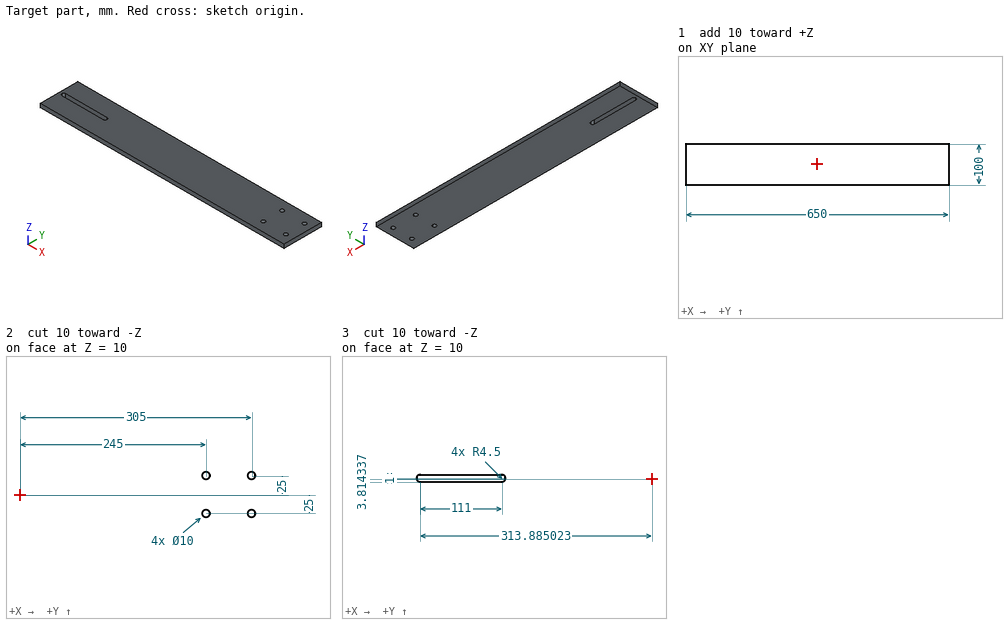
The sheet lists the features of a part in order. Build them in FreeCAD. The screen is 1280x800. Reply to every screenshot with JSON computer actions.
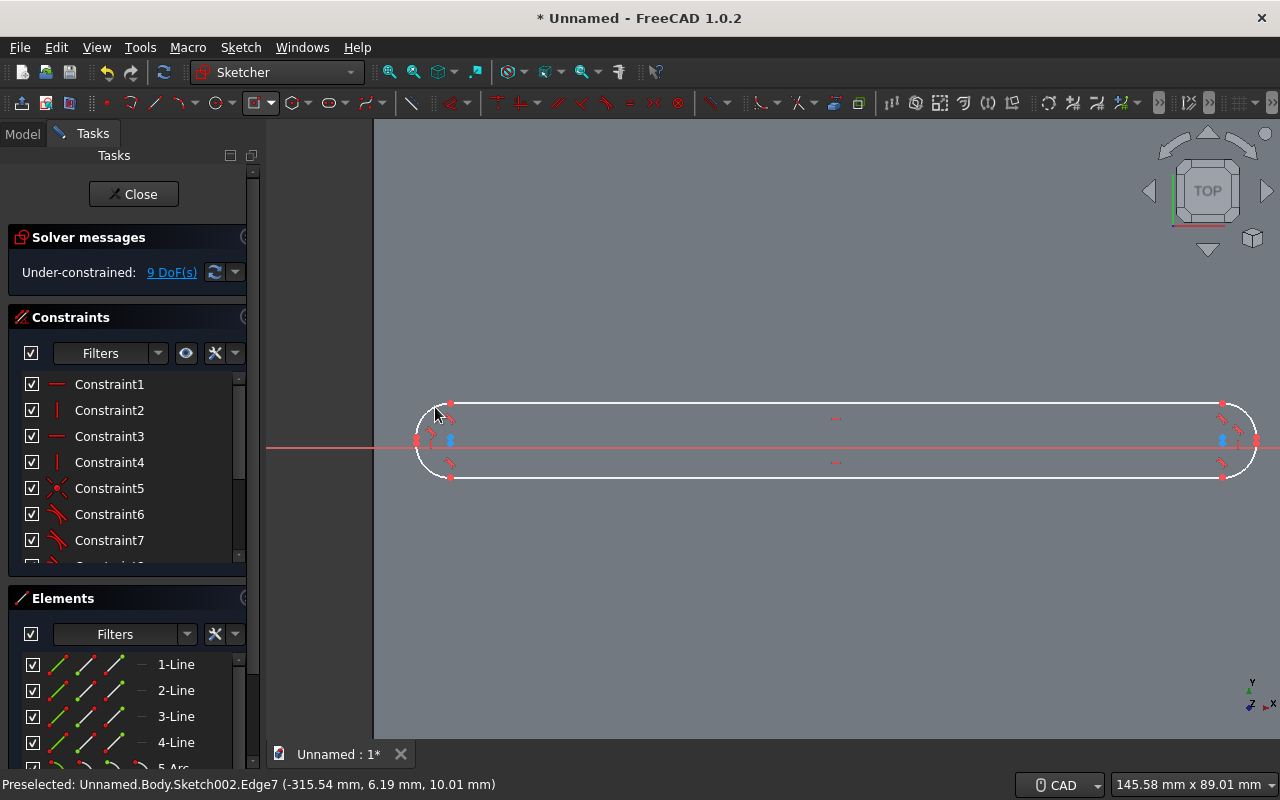
{"action": "scroll", "coordinate": [416, 441], "scroll_direction": "up", "scroll_amount": 8}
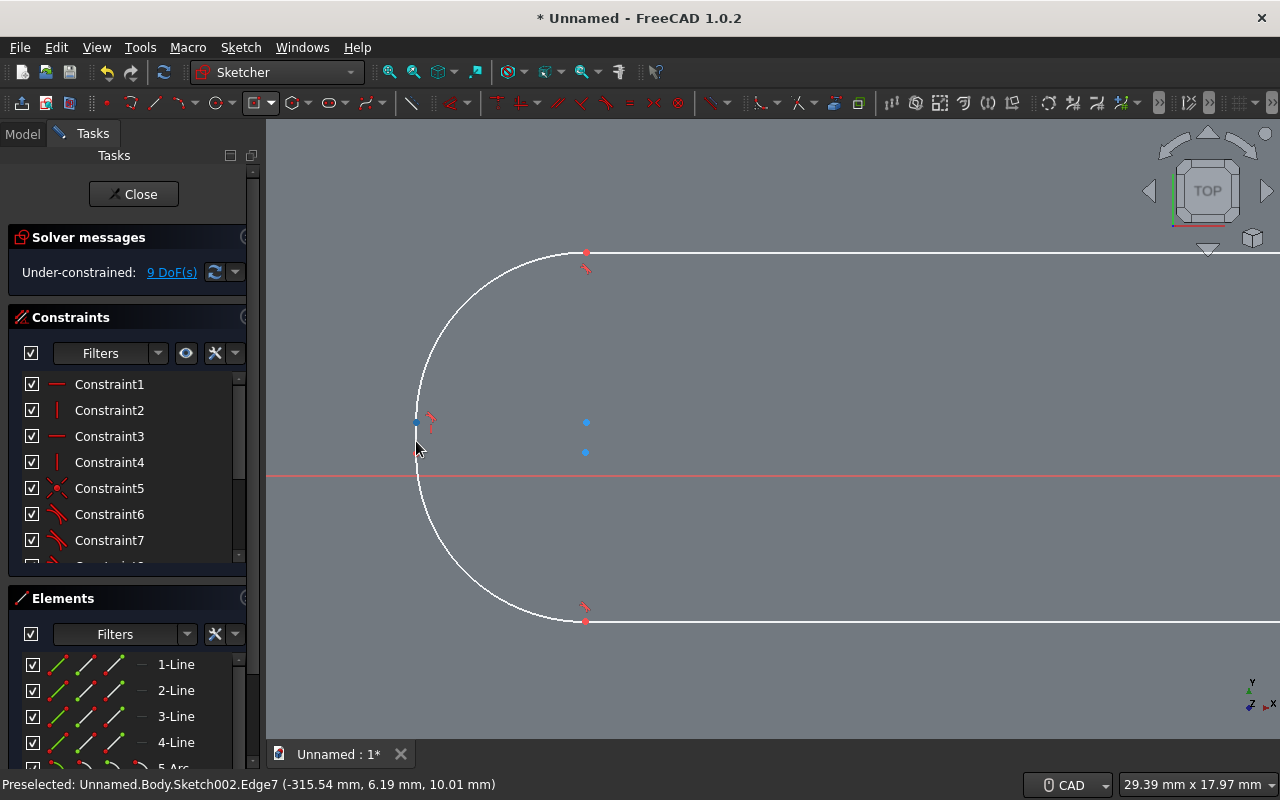
{"action": "left_click", "coordinate": [416, 438]}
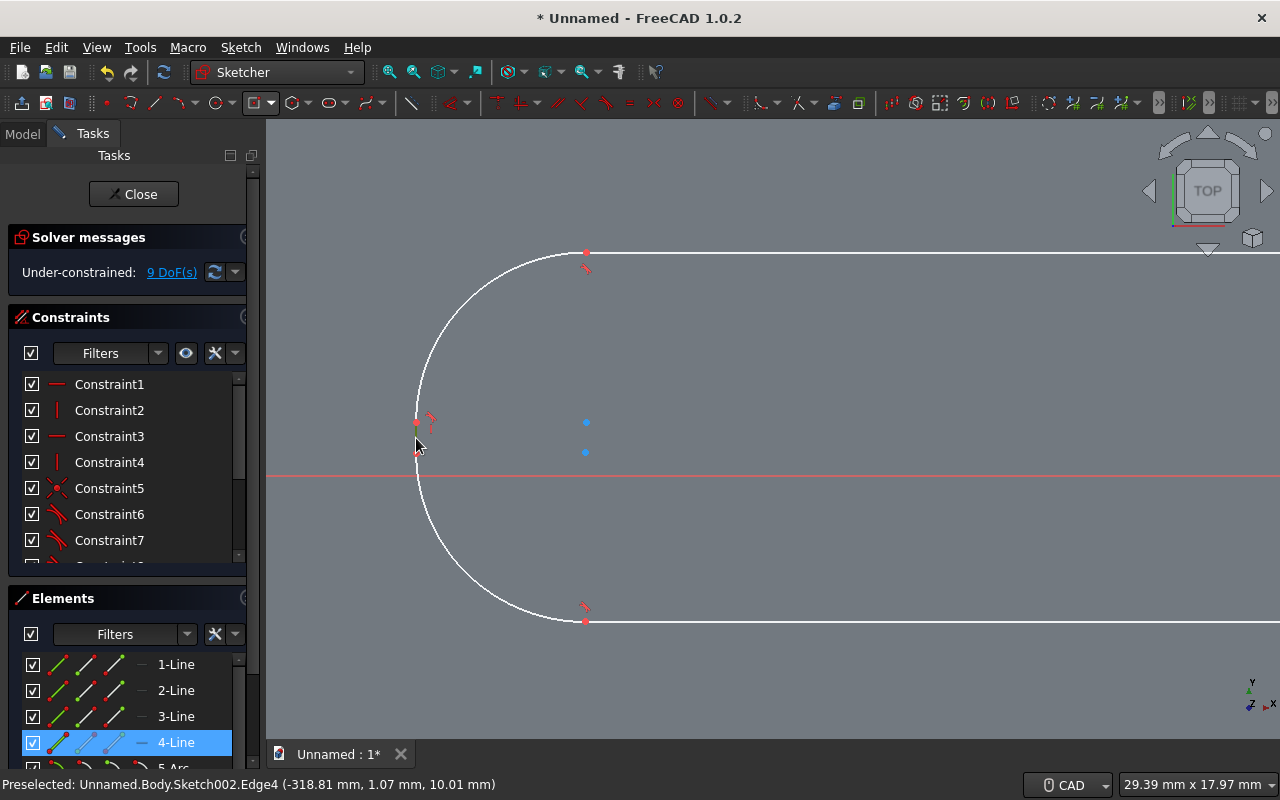
{"action": "scroll", "coordinate": [423, 428], "scroll_direction": "down", "scroll_amount": 10}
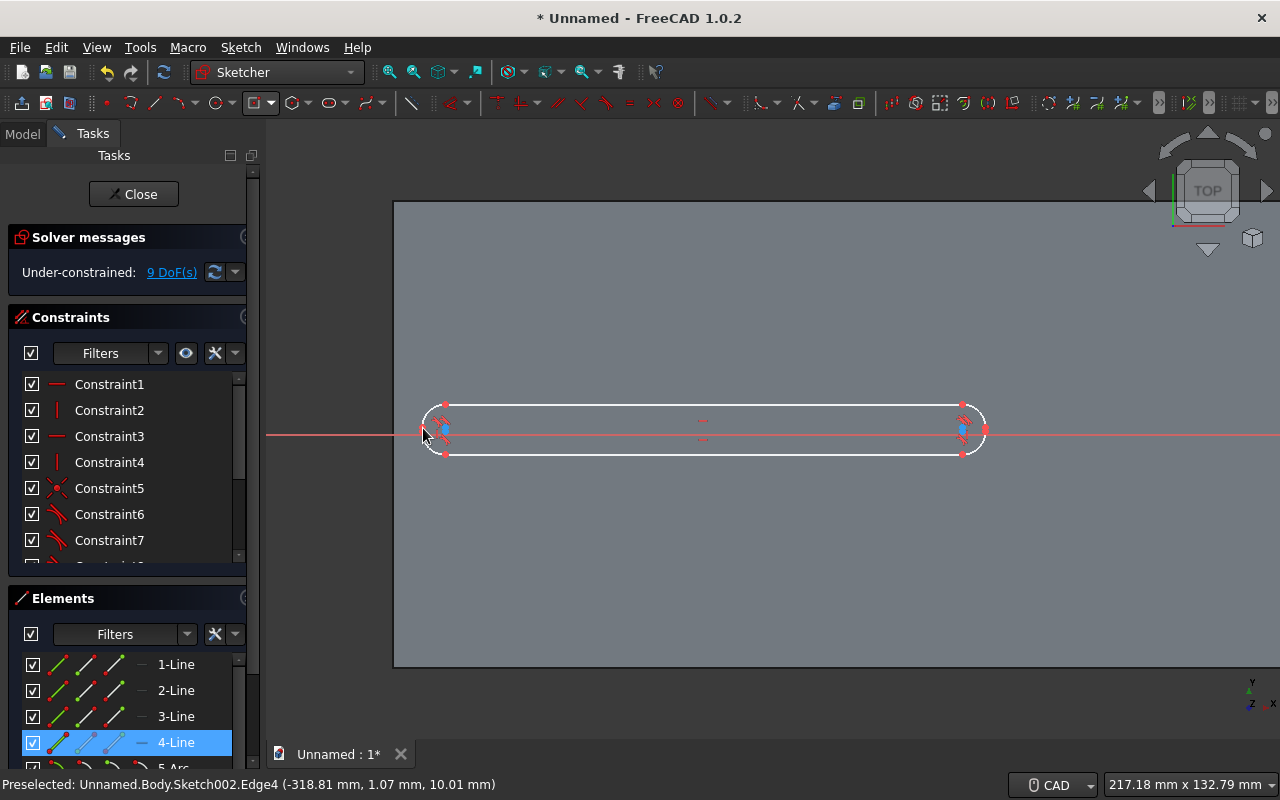
{"action": "scroll", "coordinate": [425, 442], "scroll_direction": "up", "scroll_amount": 4}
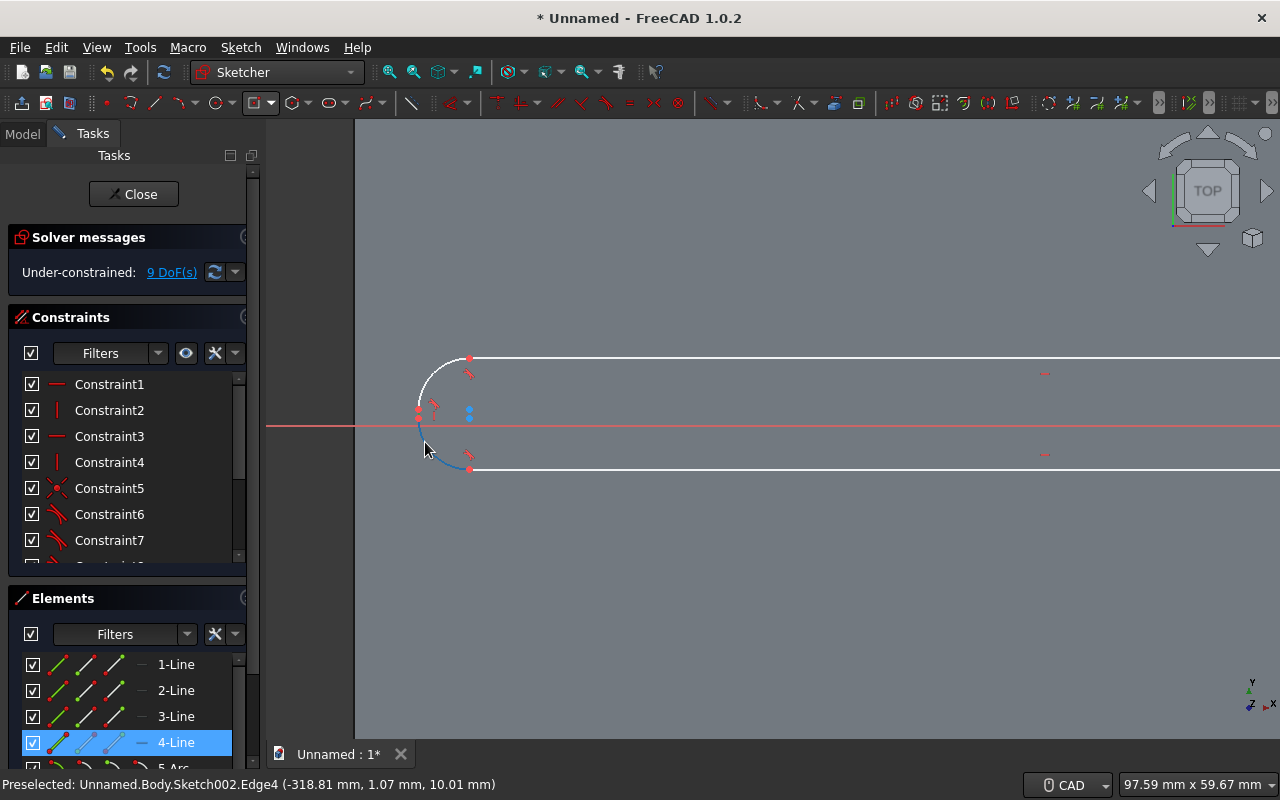
{"action": "left_click", "coordinate": [424, 442]}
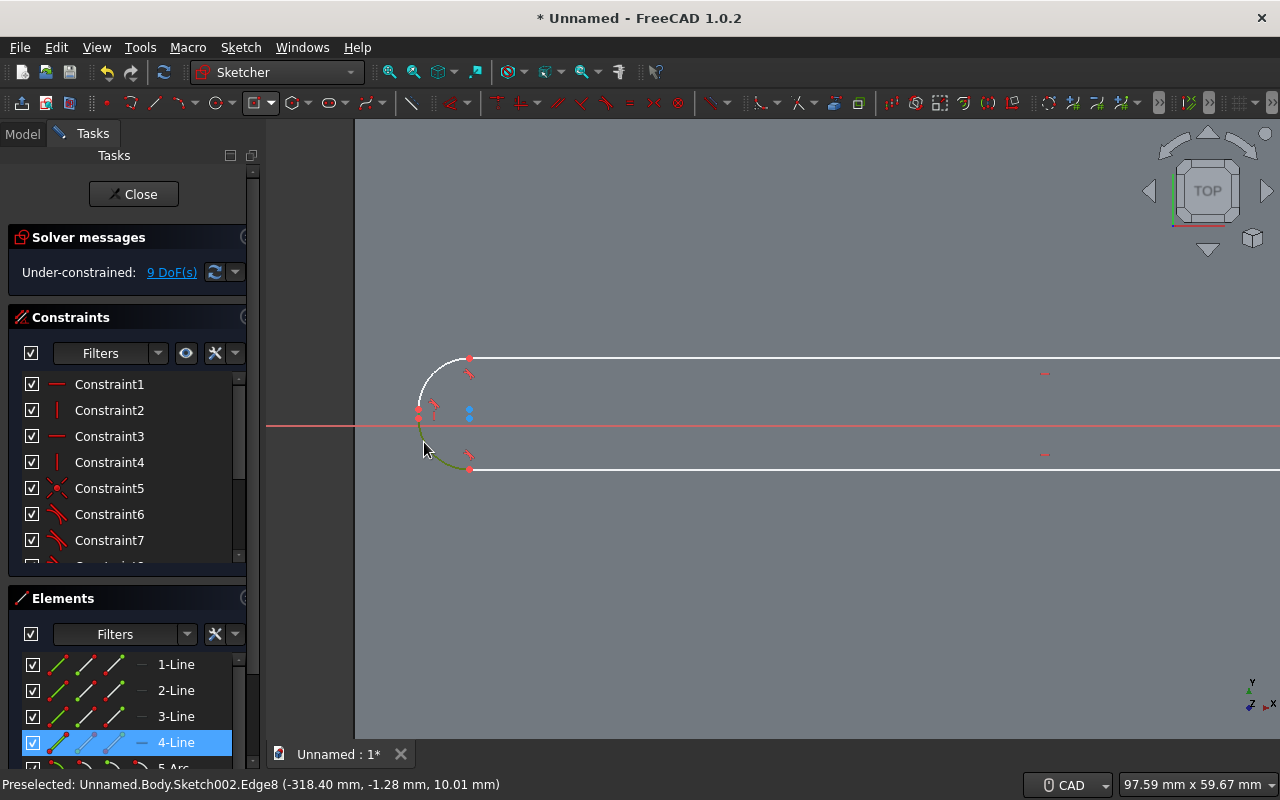
{"action": "key", "text": "t"}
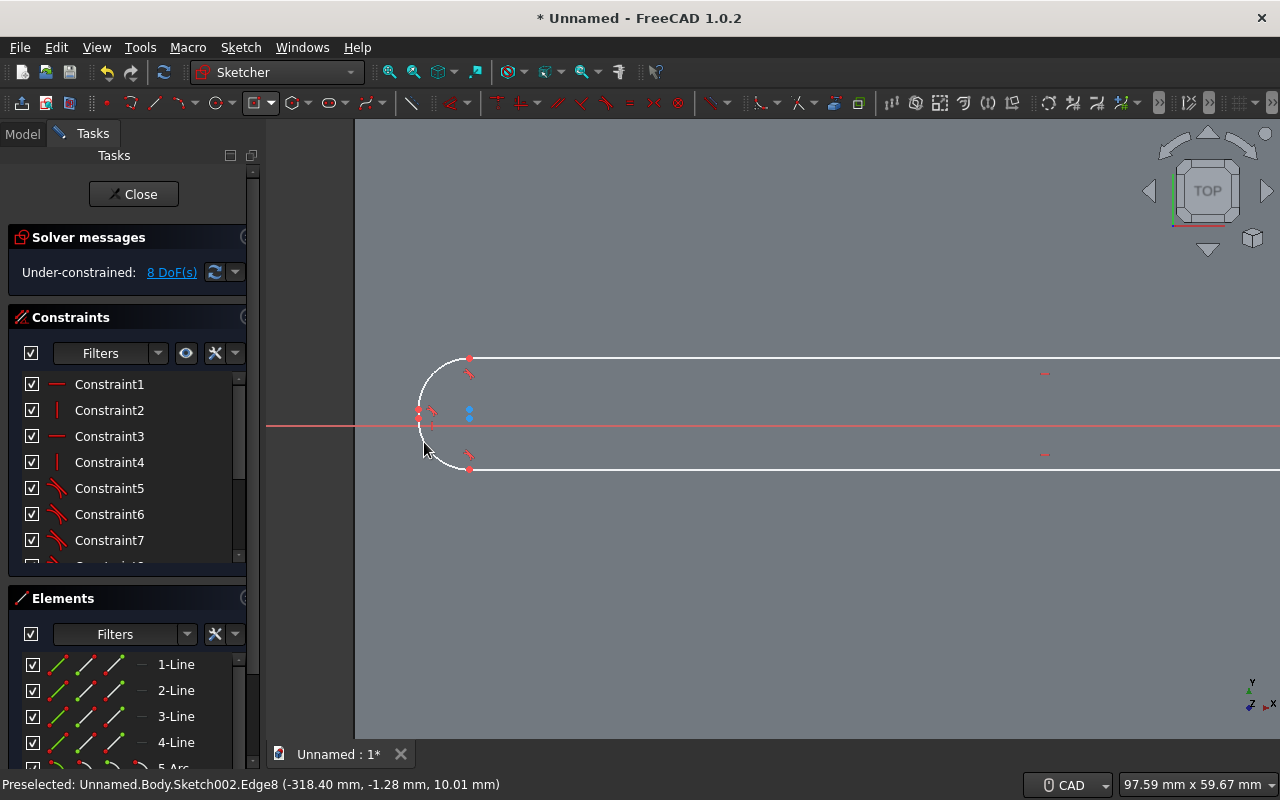
{"action": "scroll", "coordinate": [425, 442], "scroll_direction": "down", "scroll_amount": 4}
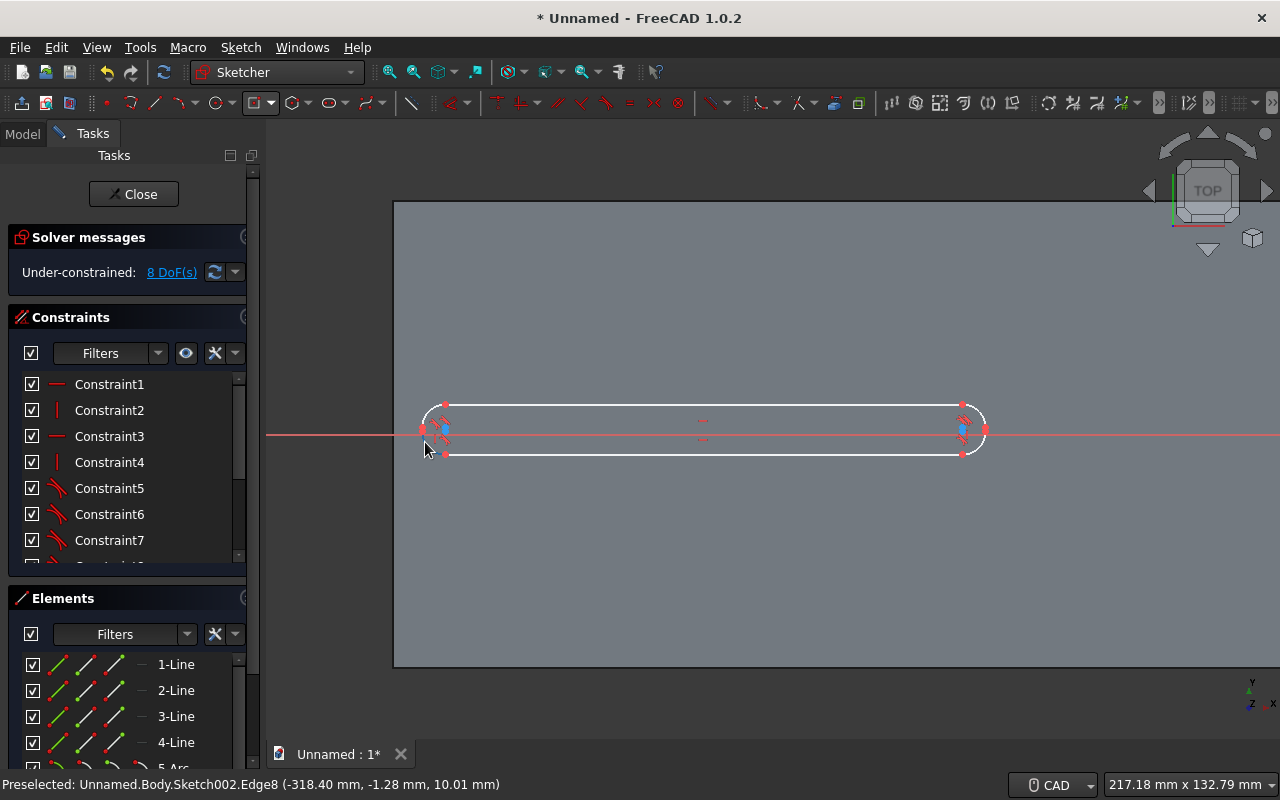
{"action": "scroll", "coordinate": [973, 452], "scroll_direction": "up", "scroll_amount": 2}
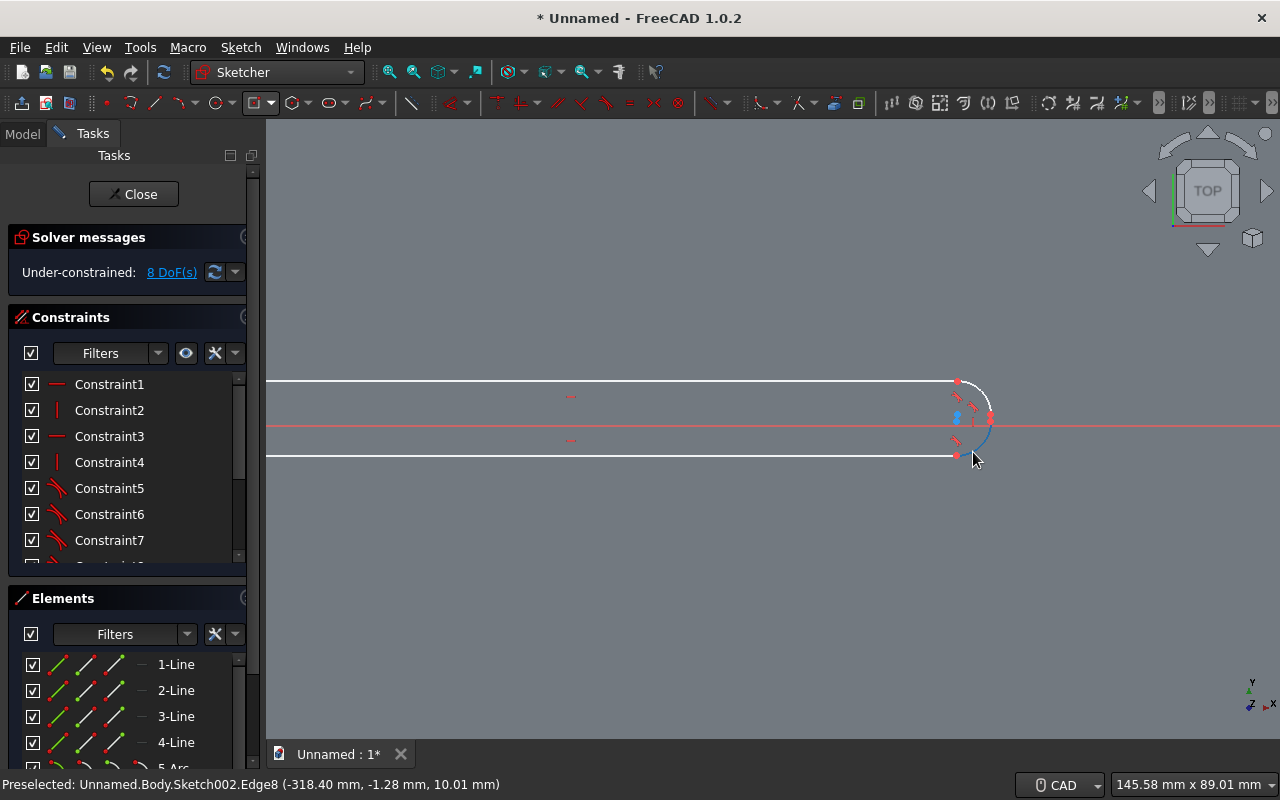
{"action": "left_click", "coordinate": [972, 452]}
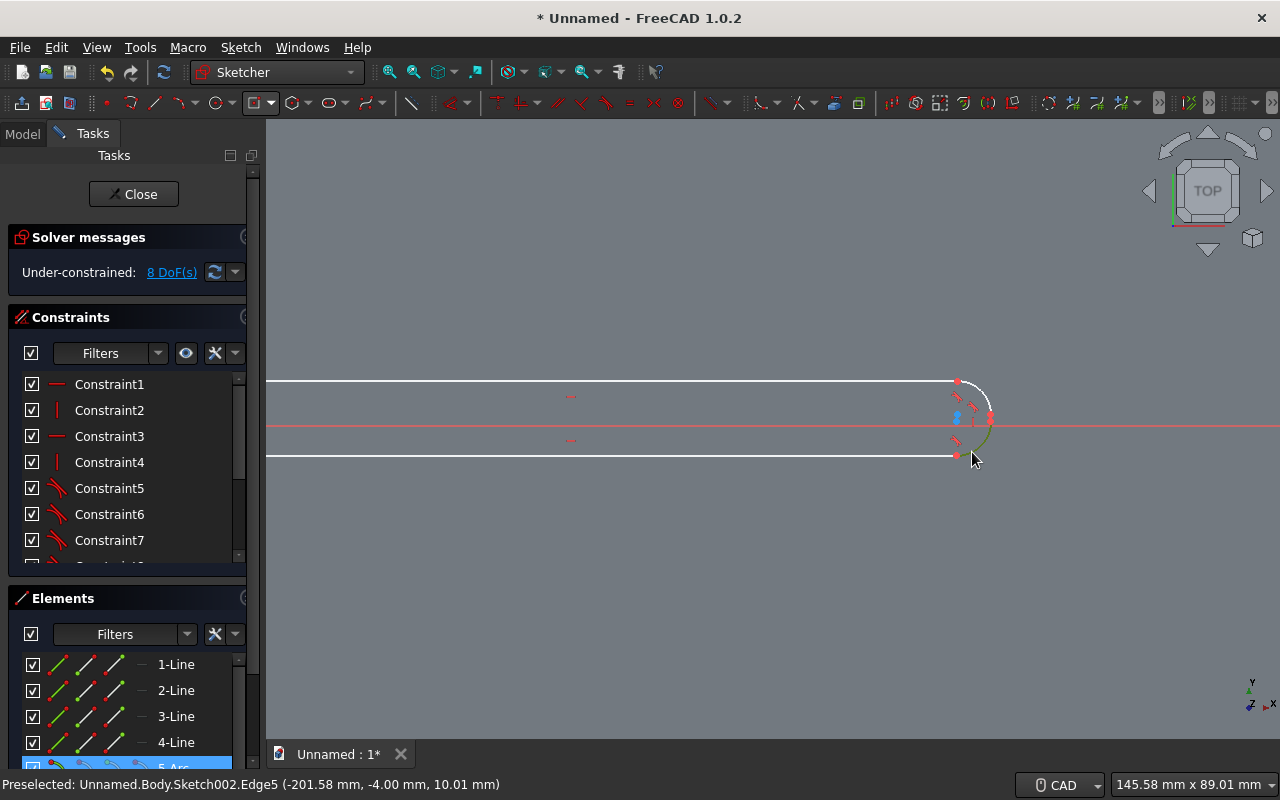
{"action": "left_click", "coordinate": [987, 400]}